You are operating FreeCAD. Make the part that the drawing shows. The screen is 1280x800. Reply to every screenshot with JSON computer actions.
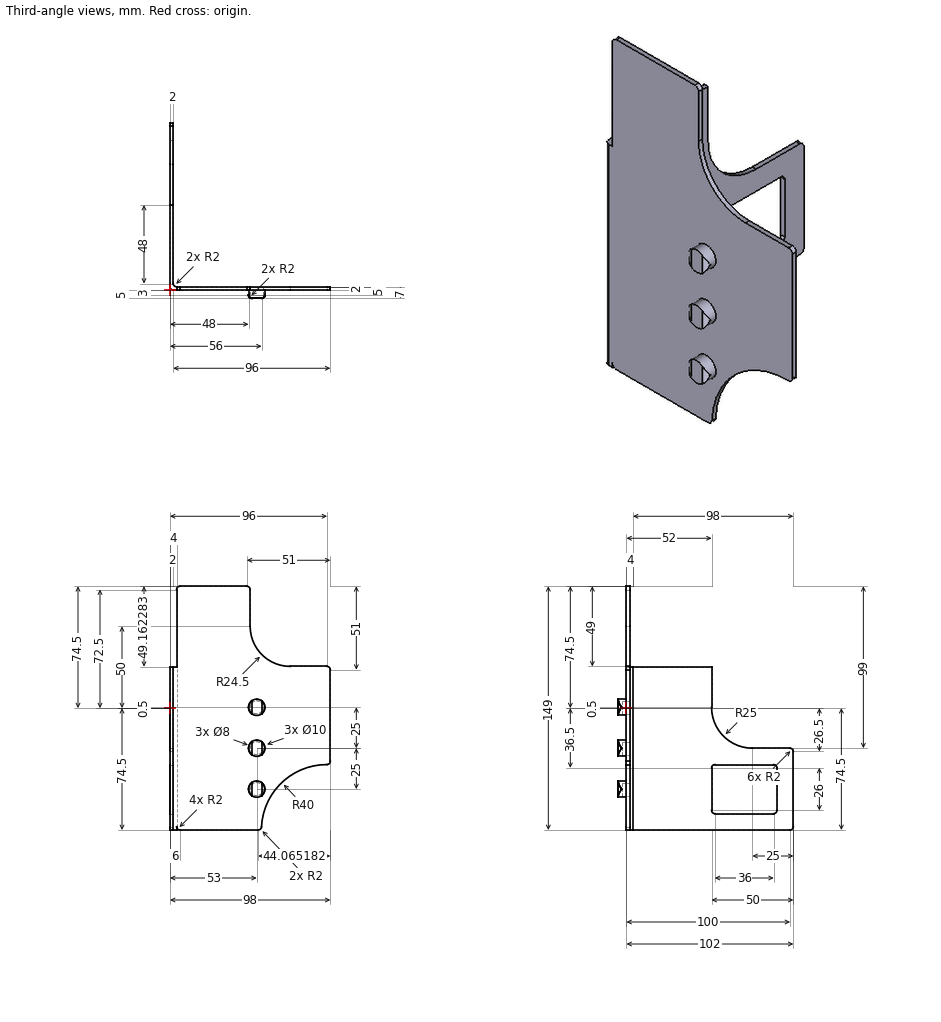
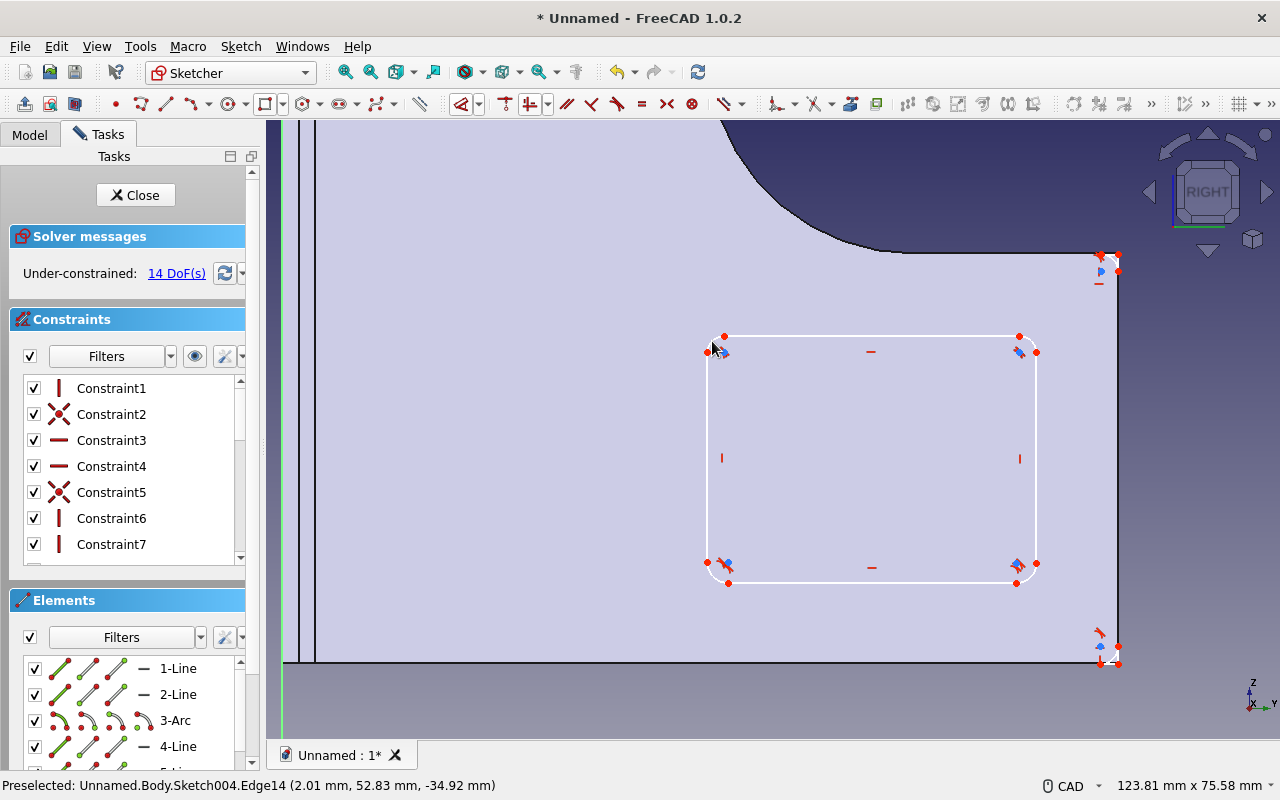
{"action": "scroll", "coordinate": [1113, 260], "scroll_direction": "up", "scroll_amount": 6}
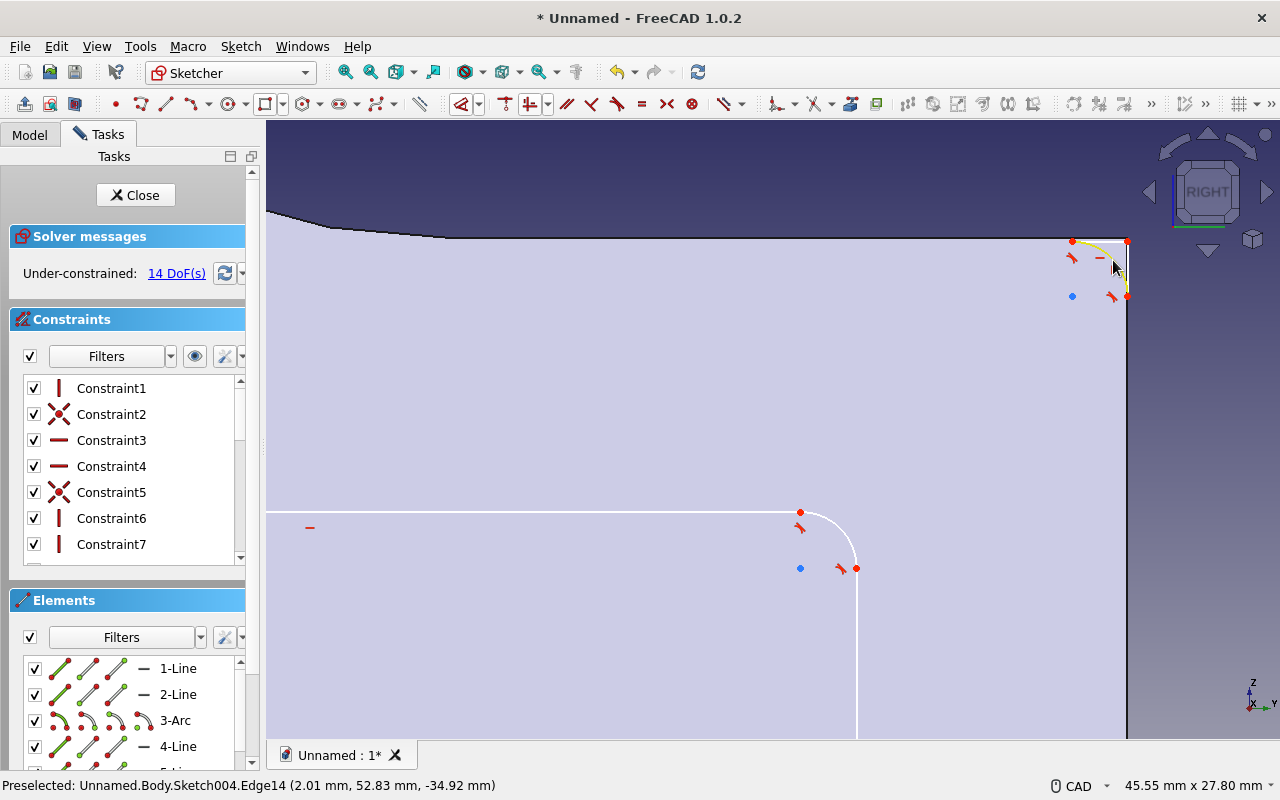
{"action": "left_click", "coordinate": [1112, 258]}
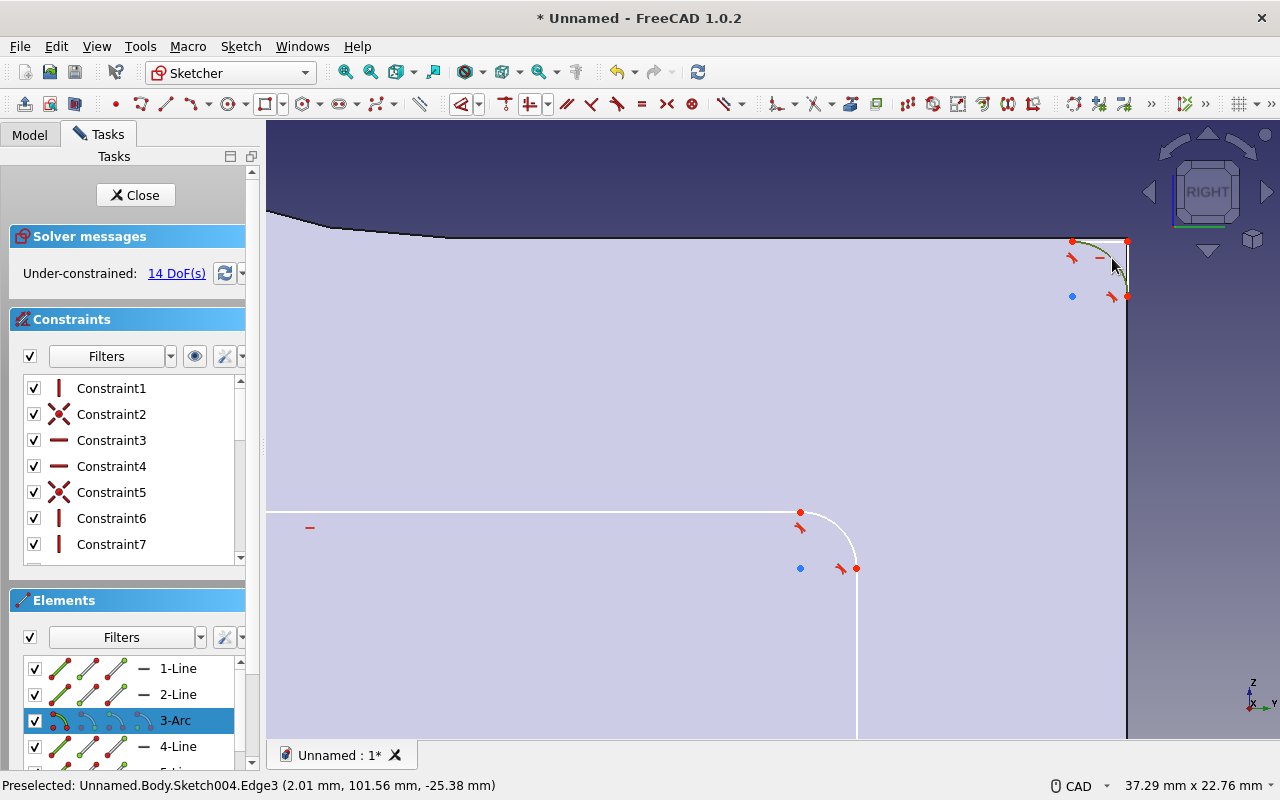
{"action": "scroll", "coordinate": [948, 390], "scroll_direction": "down", "scroll_amount": 8}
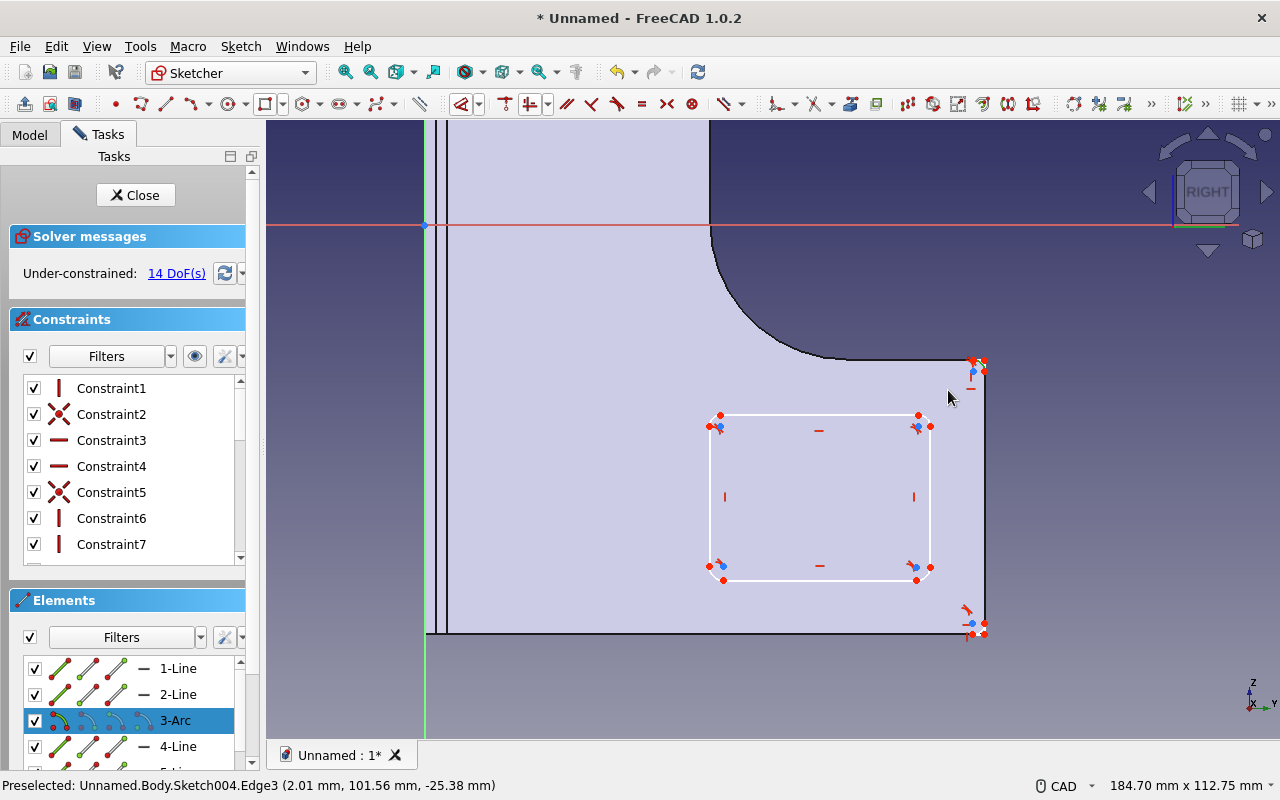
{"action": "scroll", "coordinate": [981, 632], "scroll_direction": "up", "scroll_amount": 7}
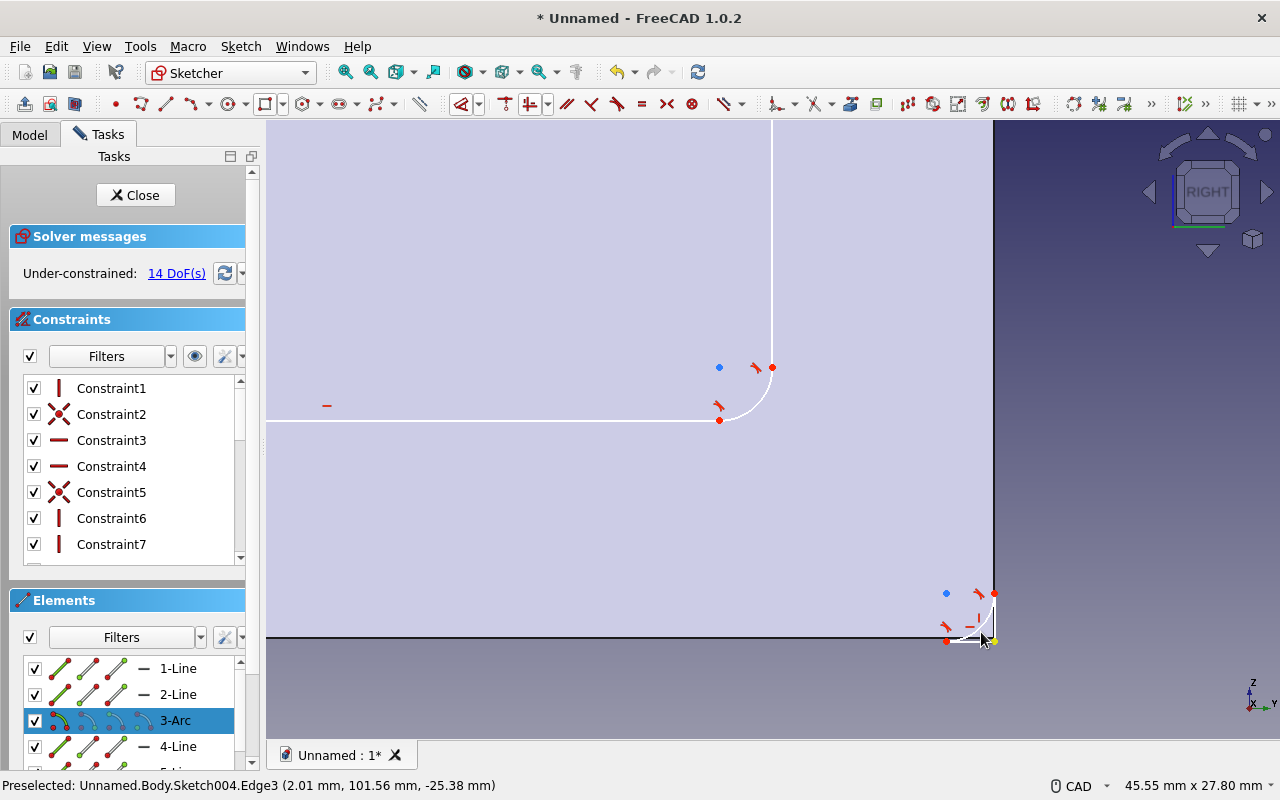
{"action": "left_click", "coordinate": [980, 628]}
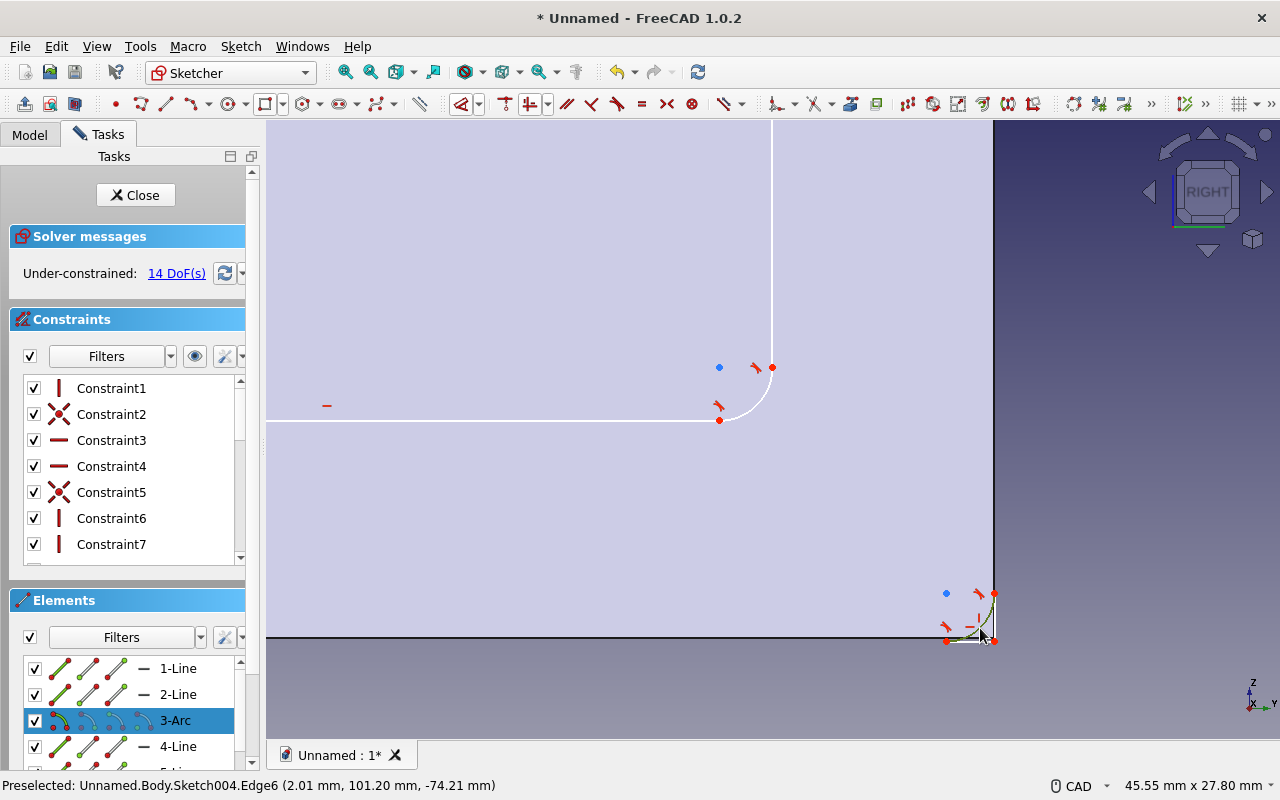
{"action": "scroll", "coordinate": [981, 633], "scroll_direction": "down", "scroll_amount": 7}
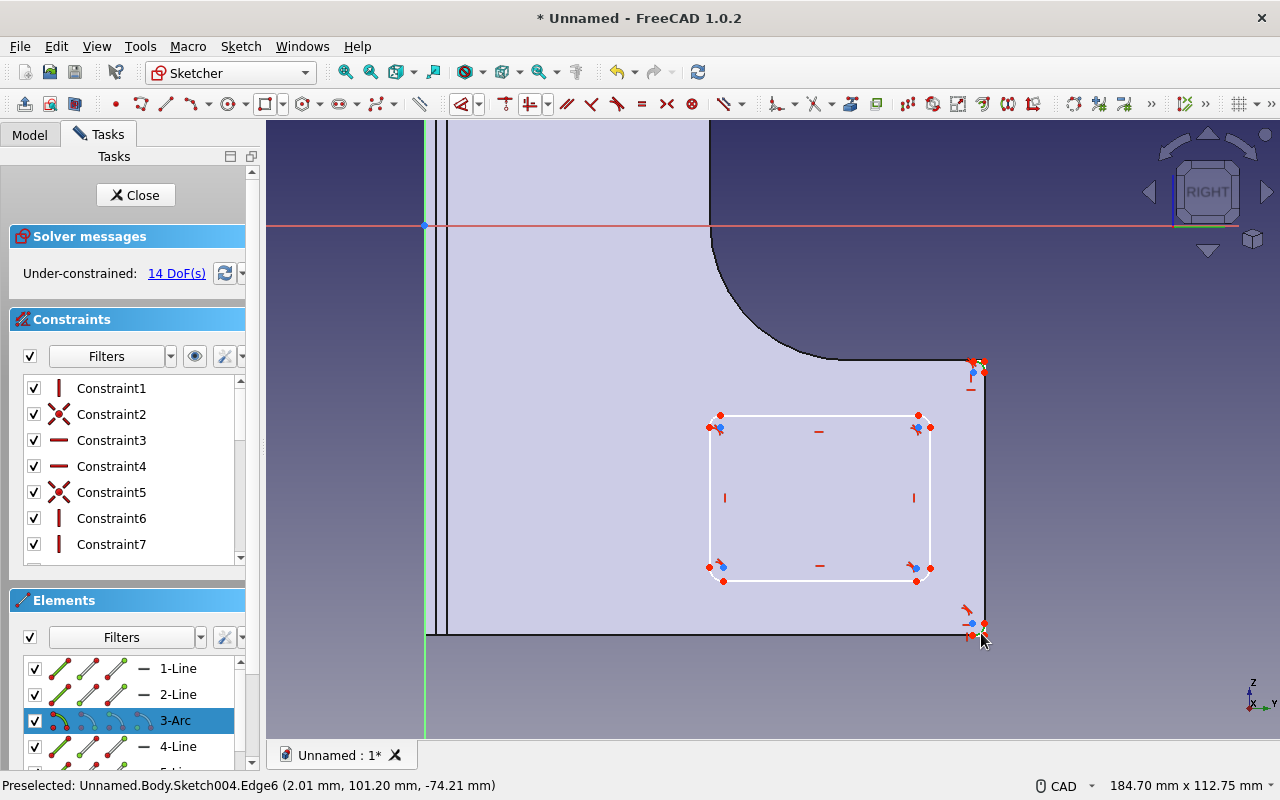
{"action": "scroll", "coordinate": [711, 574], "scroll_direction": "up", "scroll_amount": 4}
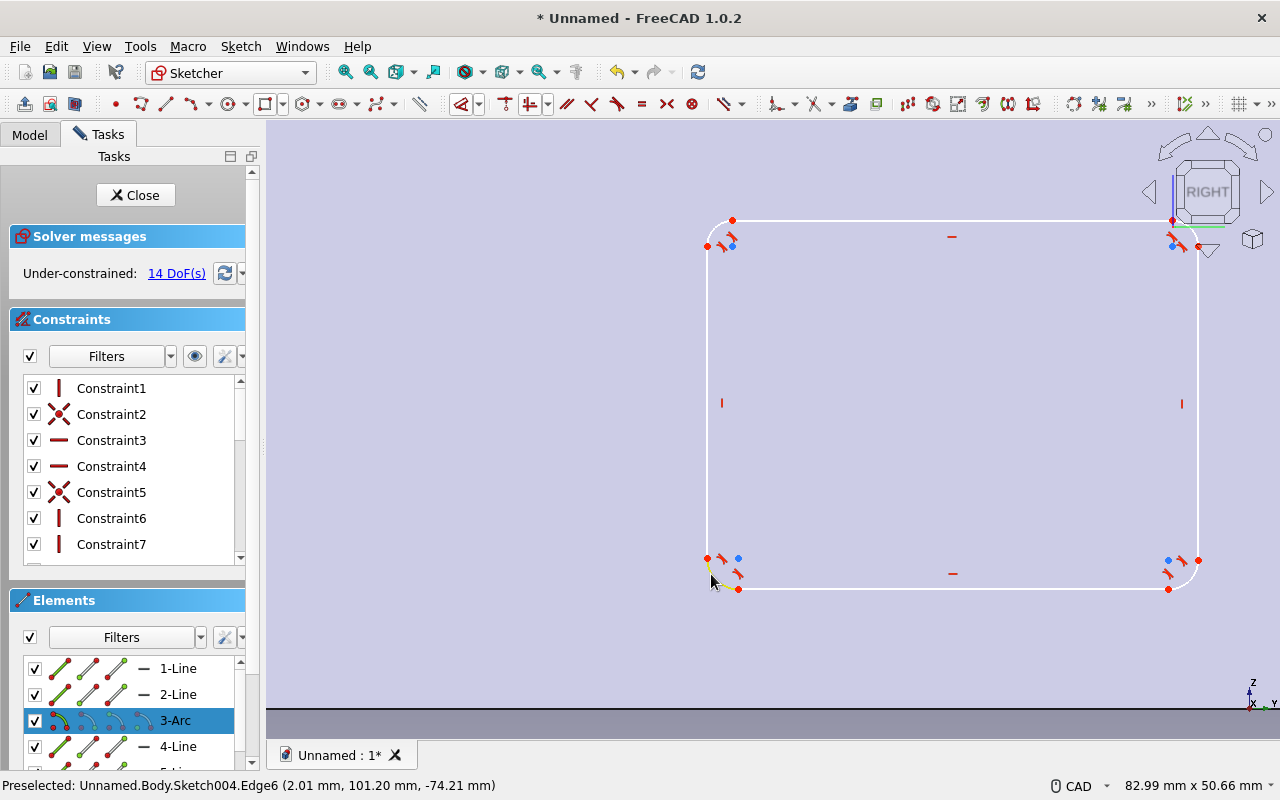
{"action": "left_click", "coordinate": [711, 572]}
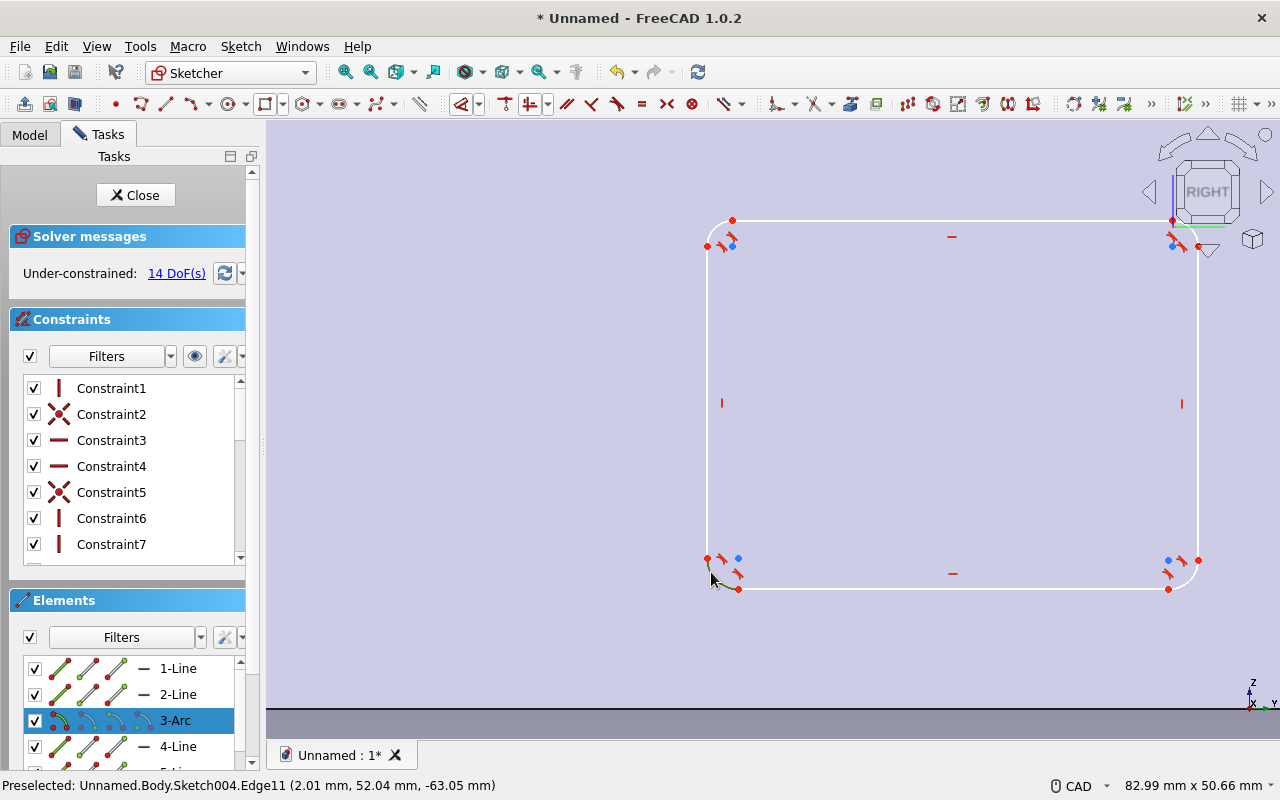
{"action": "scroll", "coordinate": [711, 573], "scroll_direction": "down", "scroll_amount": 4}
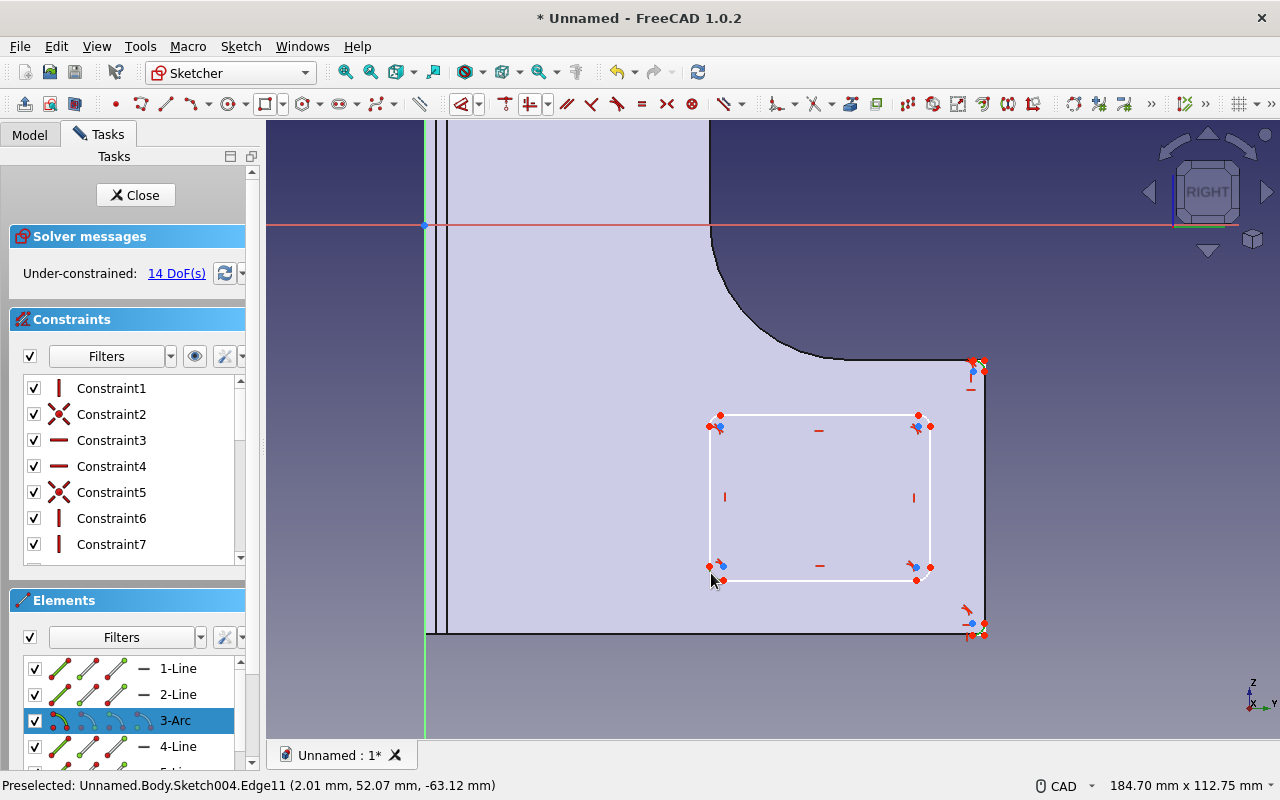
{"action": "scroll", "coordinate": [923, 579], "scroll_direction": "up", "scroll_amount": 5}